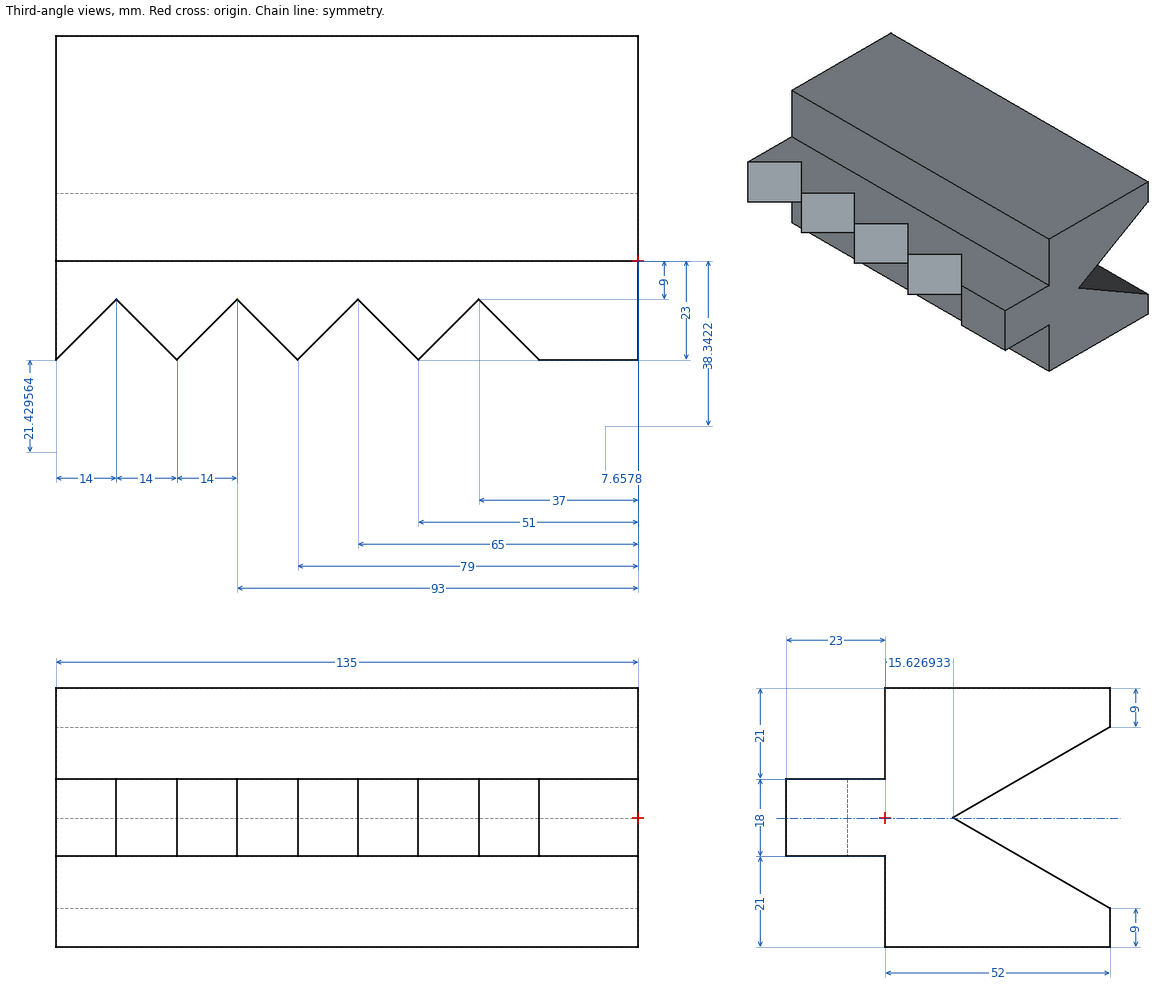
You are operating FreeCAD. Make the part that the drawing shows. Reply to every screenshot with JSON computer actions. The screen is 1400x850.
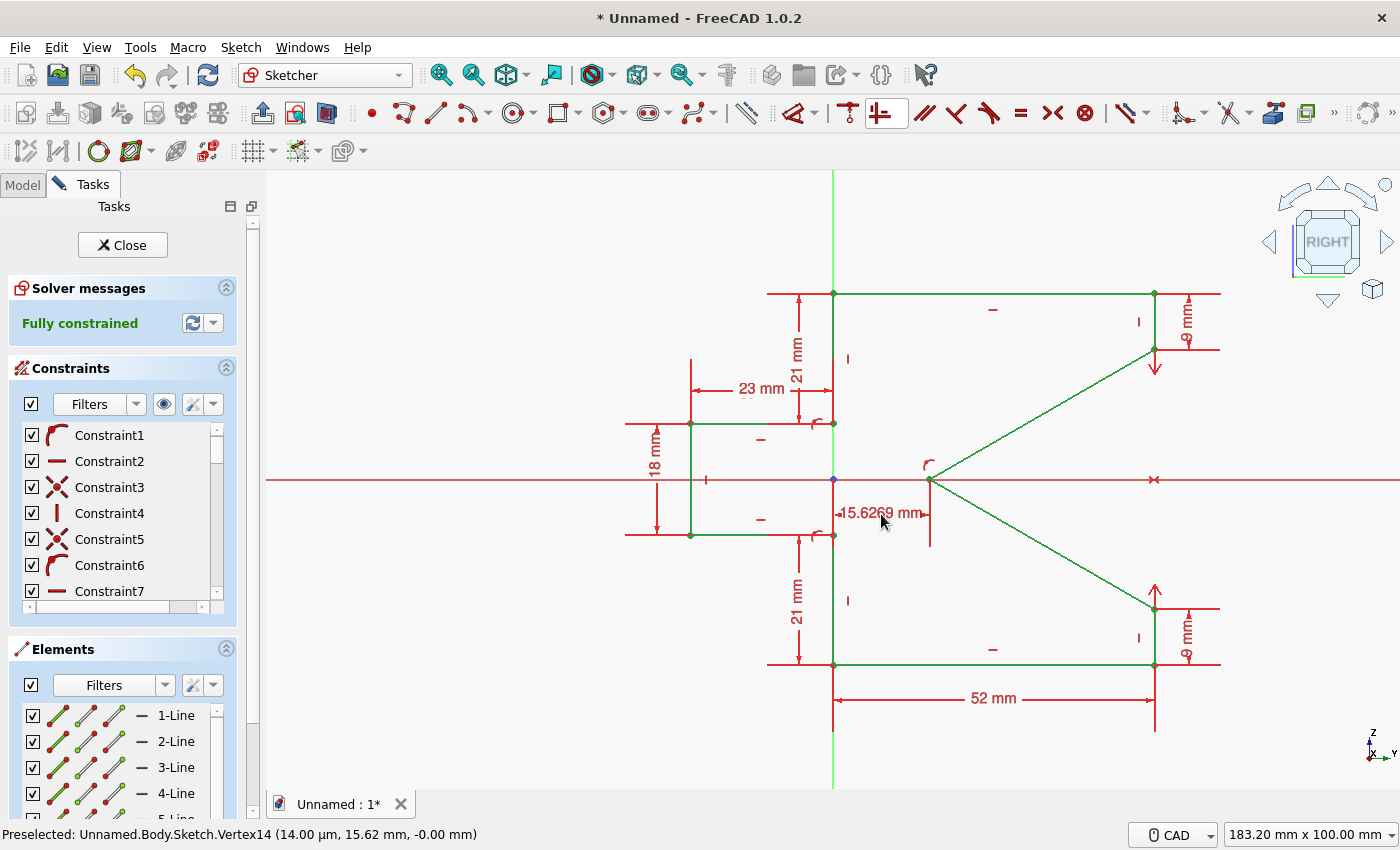
{"action": "left_click", "coordinate": [123, 245]}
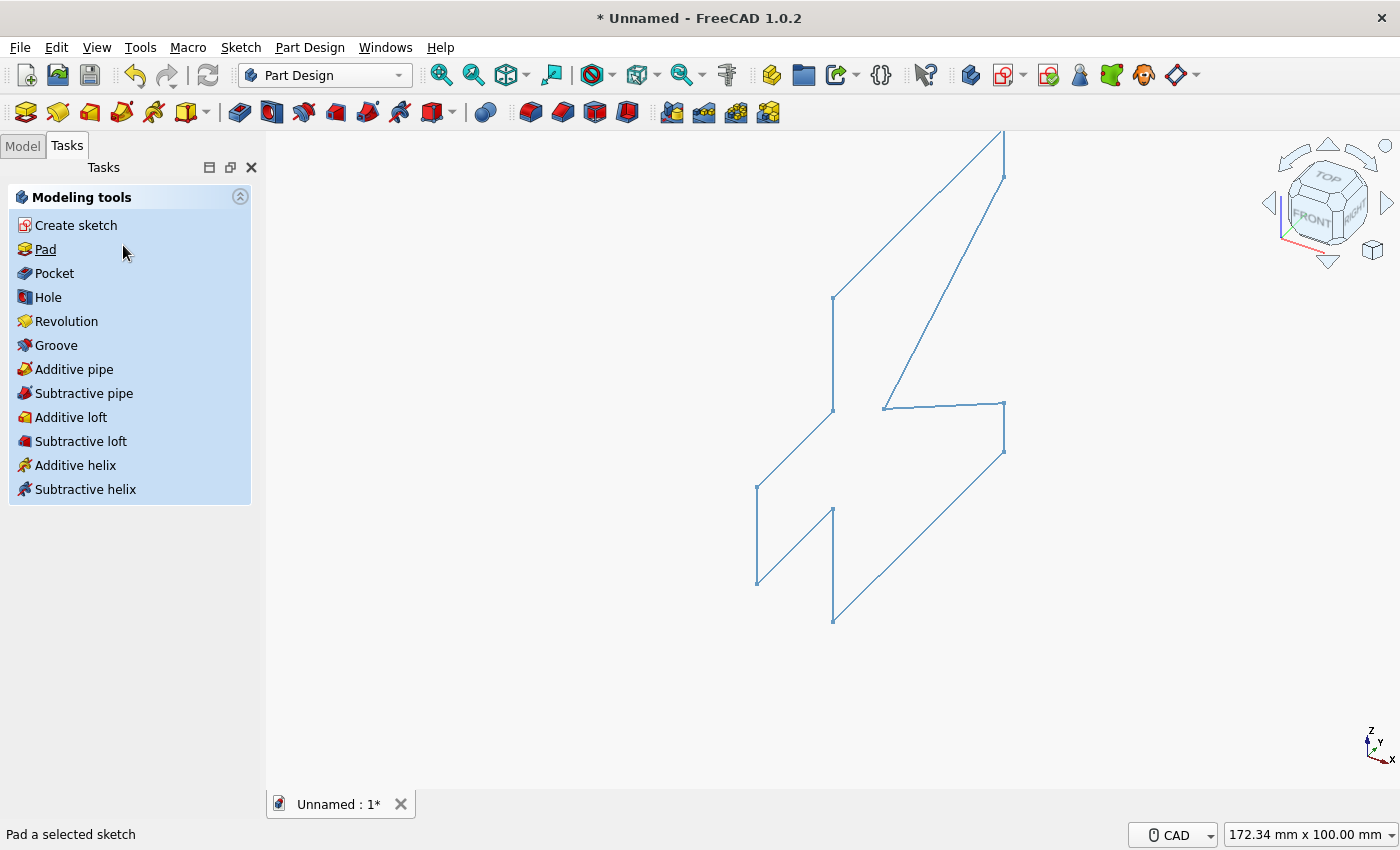
{"action": "left_click", "coordinate": [26, 112]}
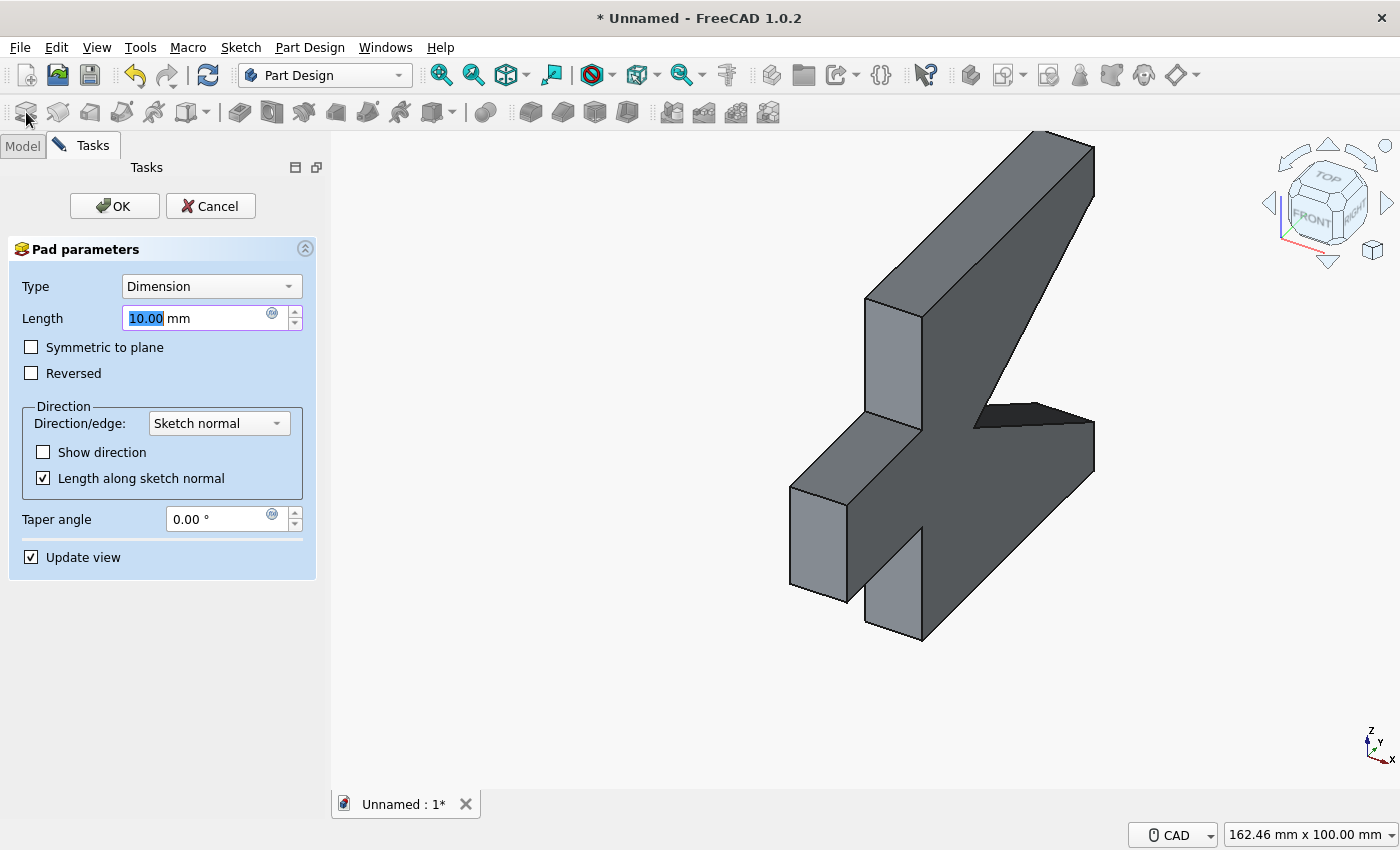
{"action": "type", "text": "135"}
{"action": "key", "text": "Tab"}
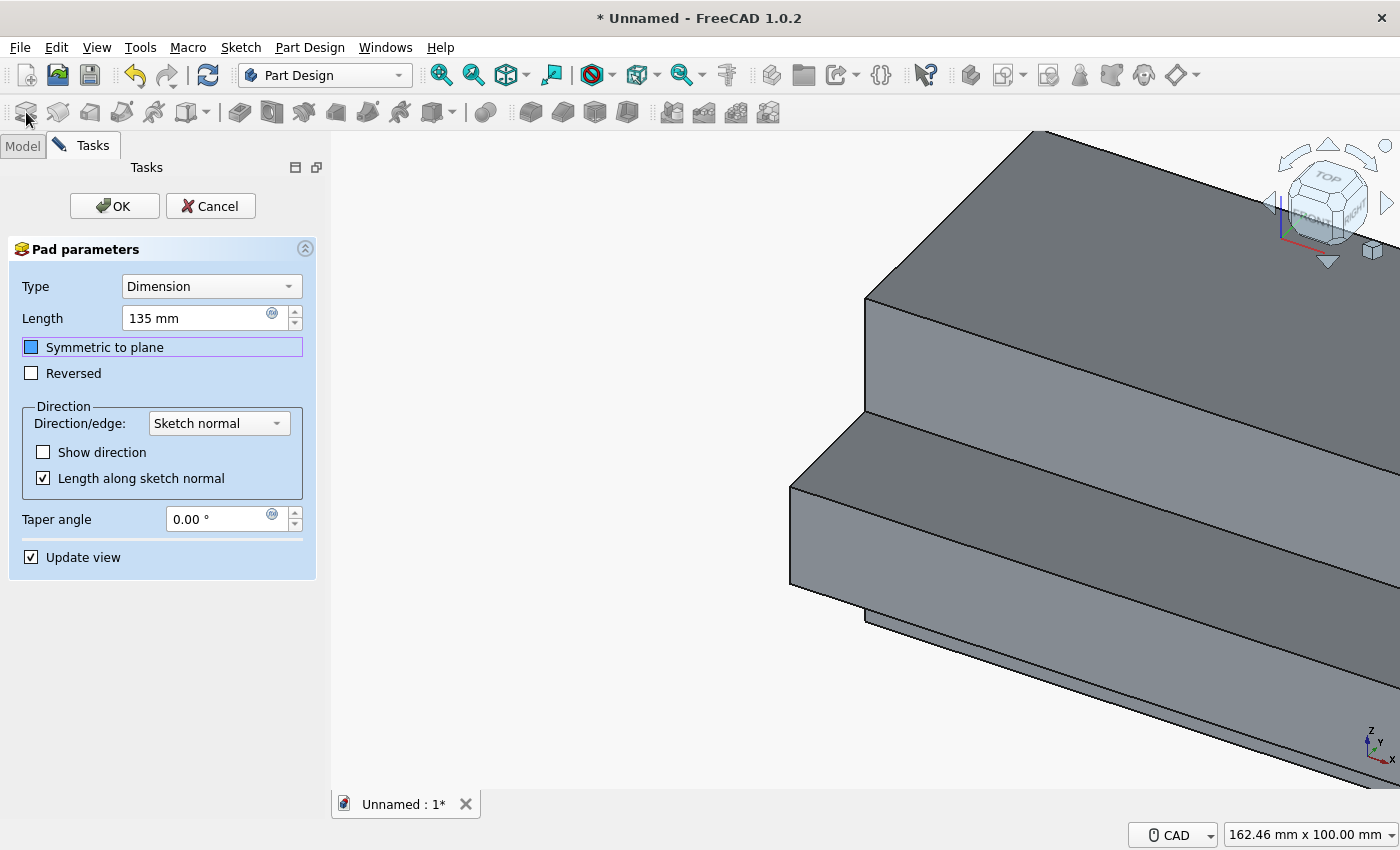
{"action": "left_click", "coordinate": [30, 373]}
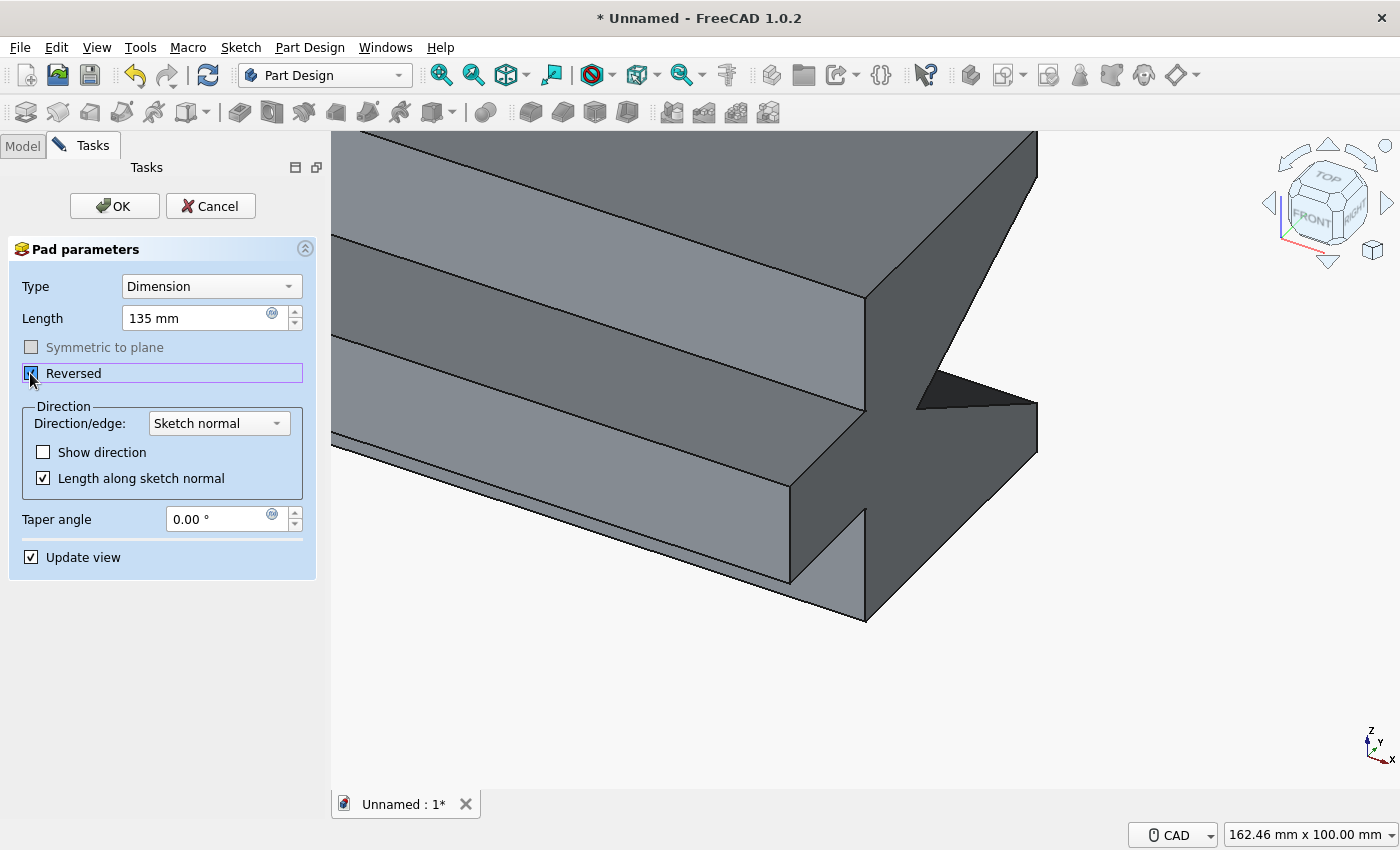
{"action": "left_click", "coordinate": [115, 206]}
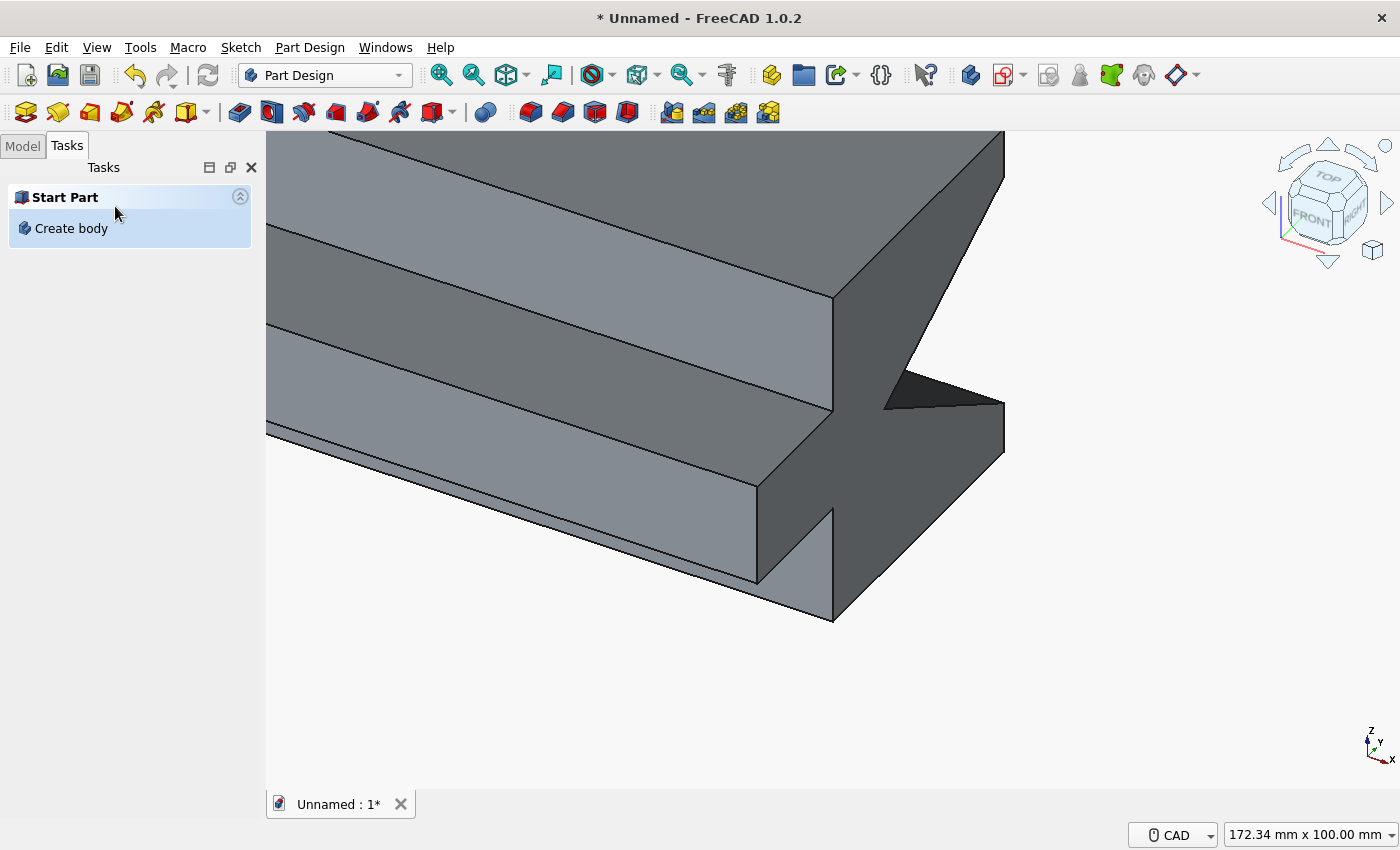
{"action": "left_click", "coordinate": [442, 76]}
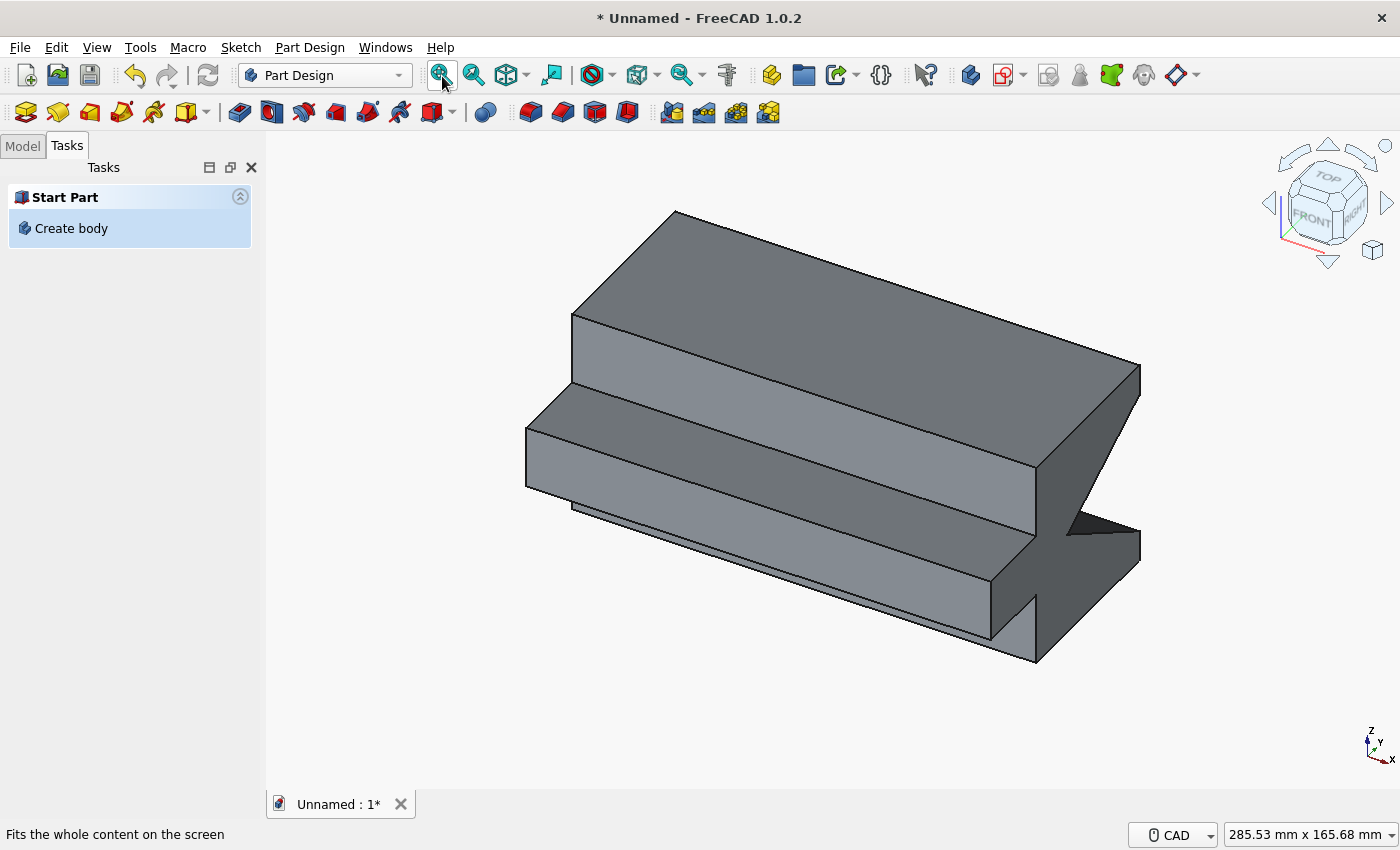
{"action": "left_click", "coordinate": [715, 459]}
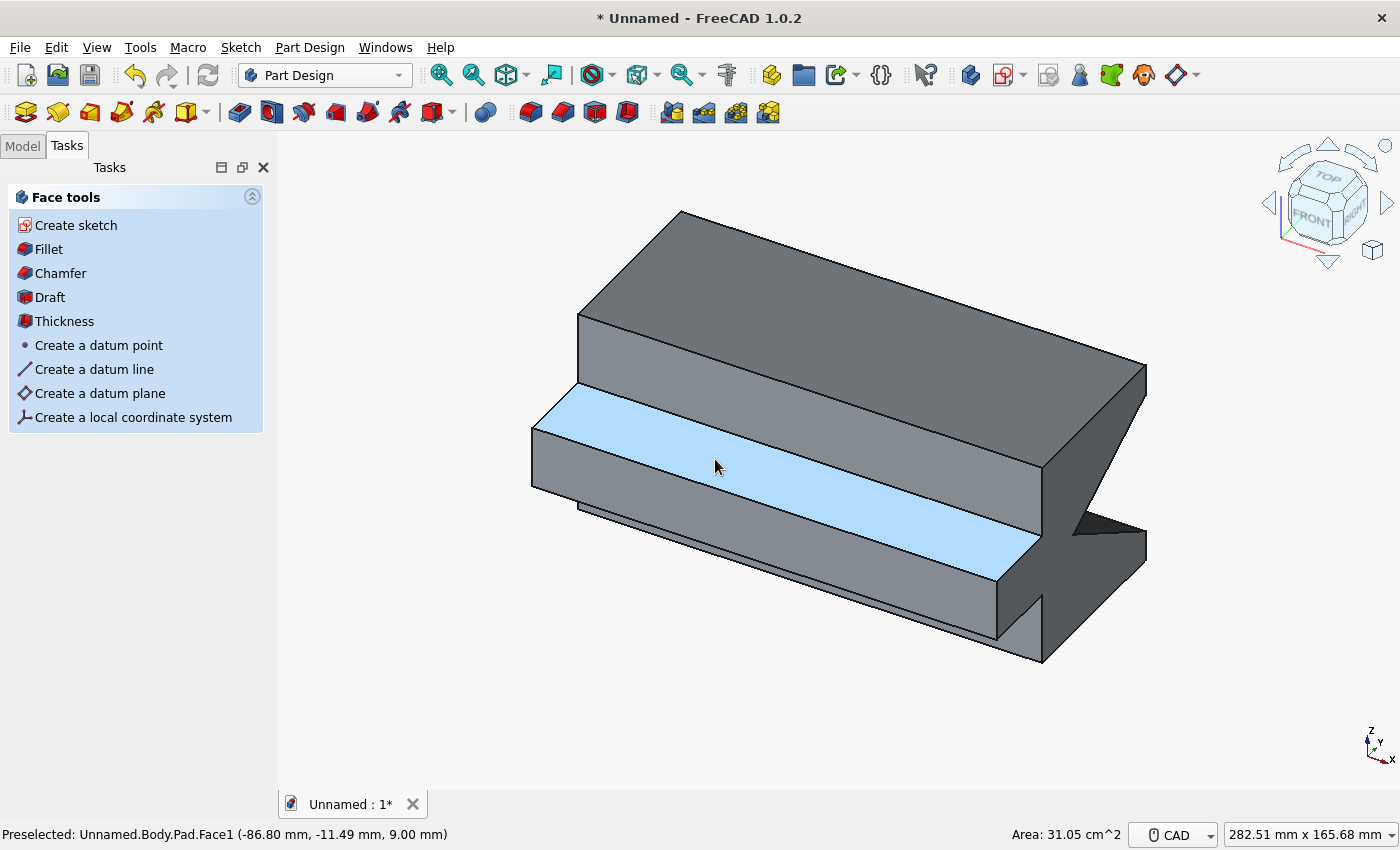
{"action": "left_click", "coordinate": [1004, 76]}